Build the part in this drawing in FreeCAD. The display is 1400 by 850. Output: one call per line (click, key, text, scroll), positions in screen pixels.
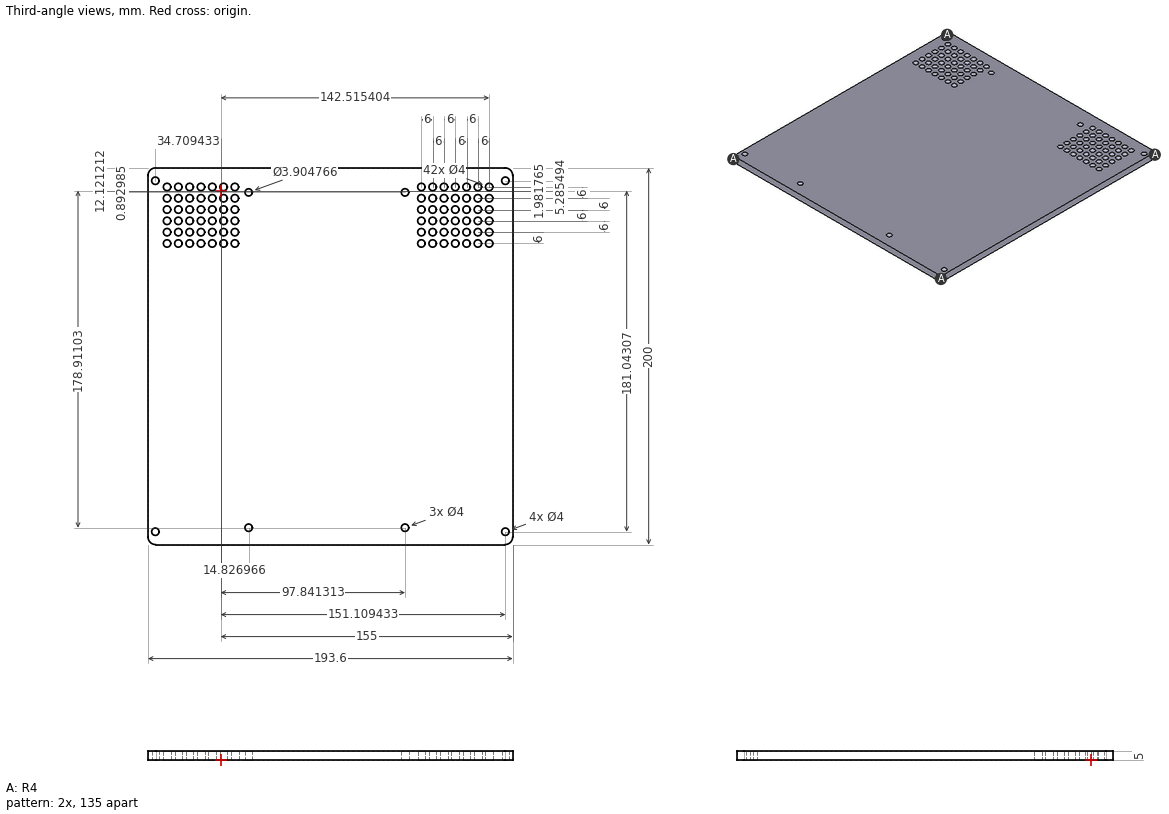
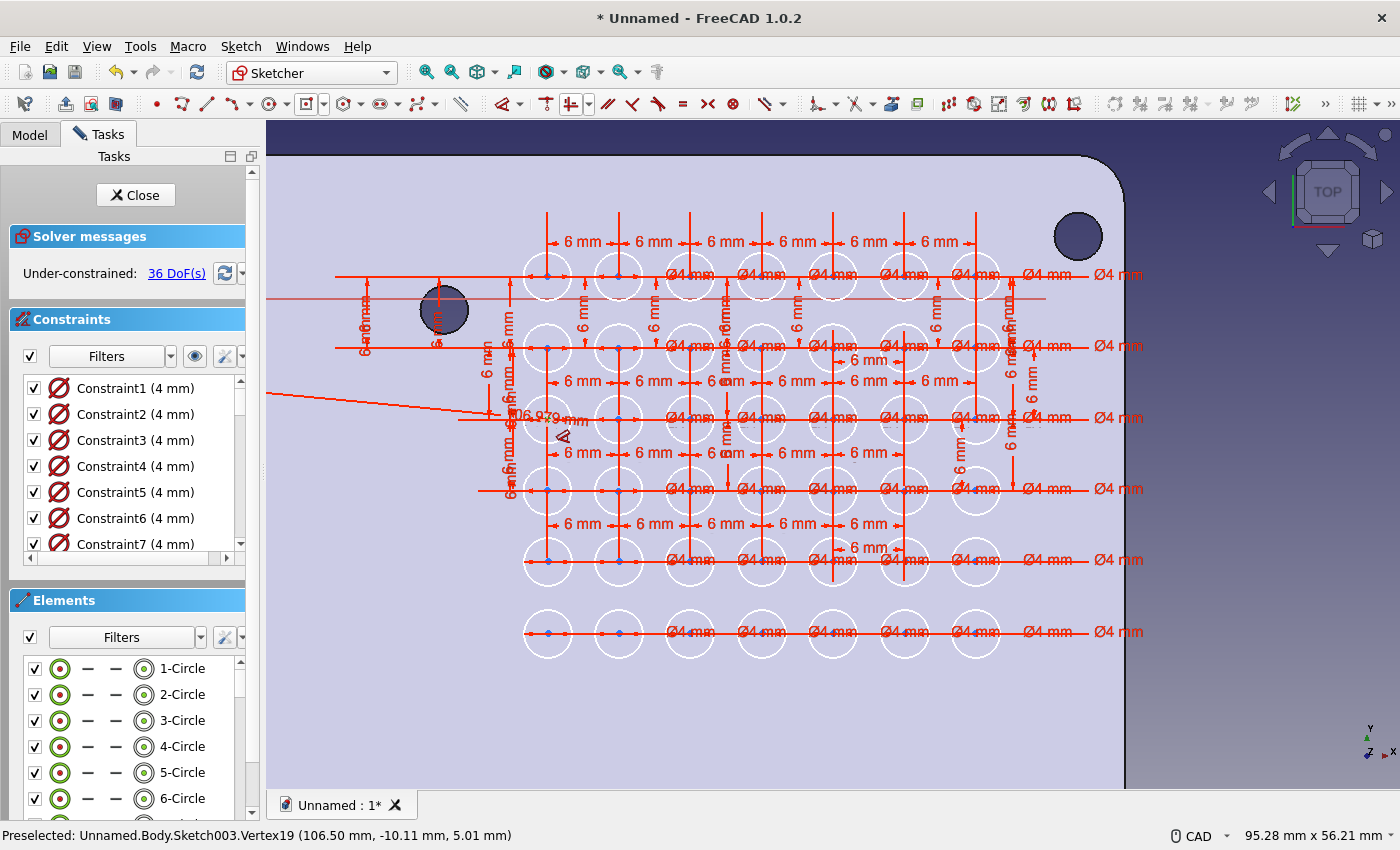
click(547, 491)
click(489, 430)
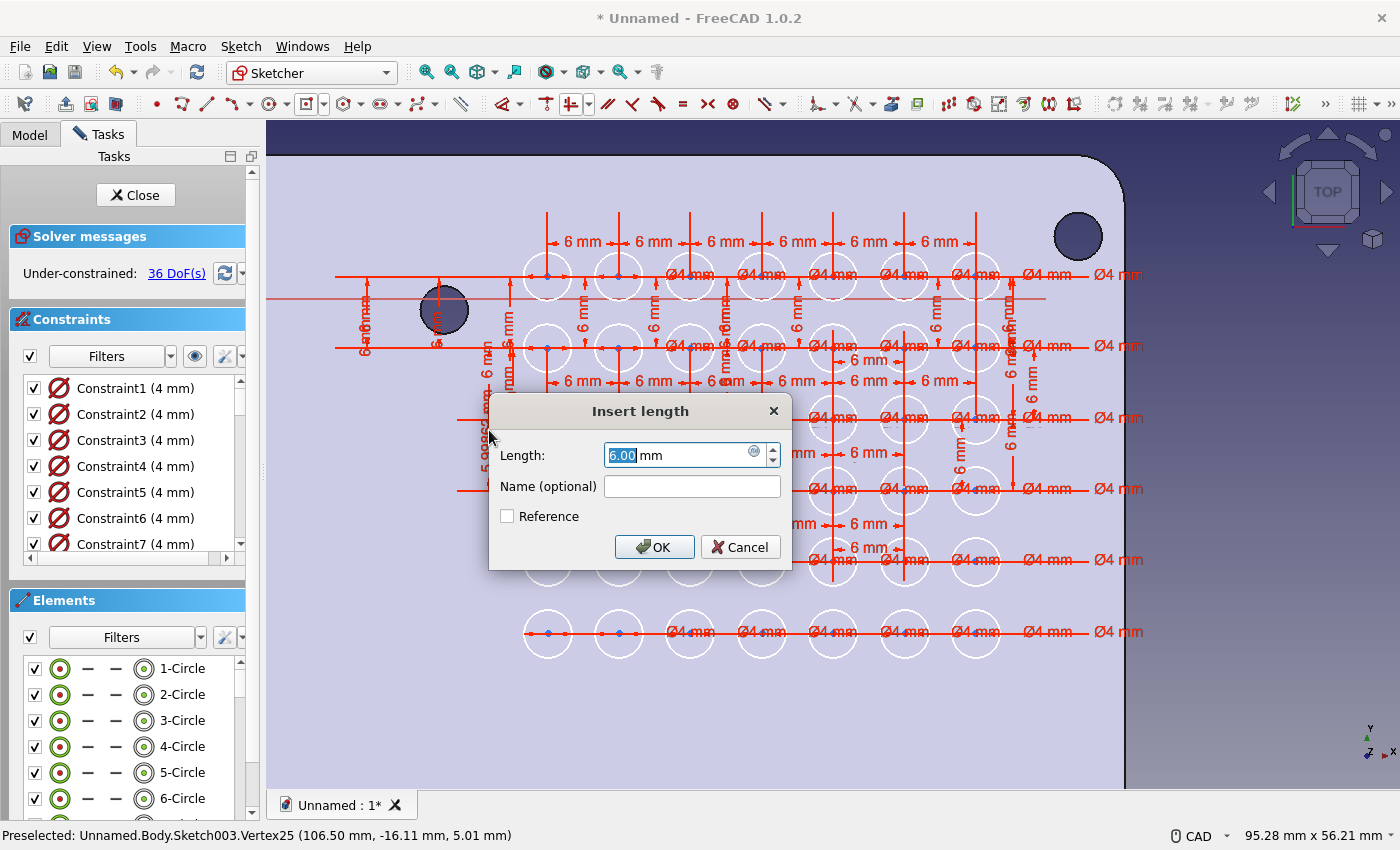
text(6)
key(Return)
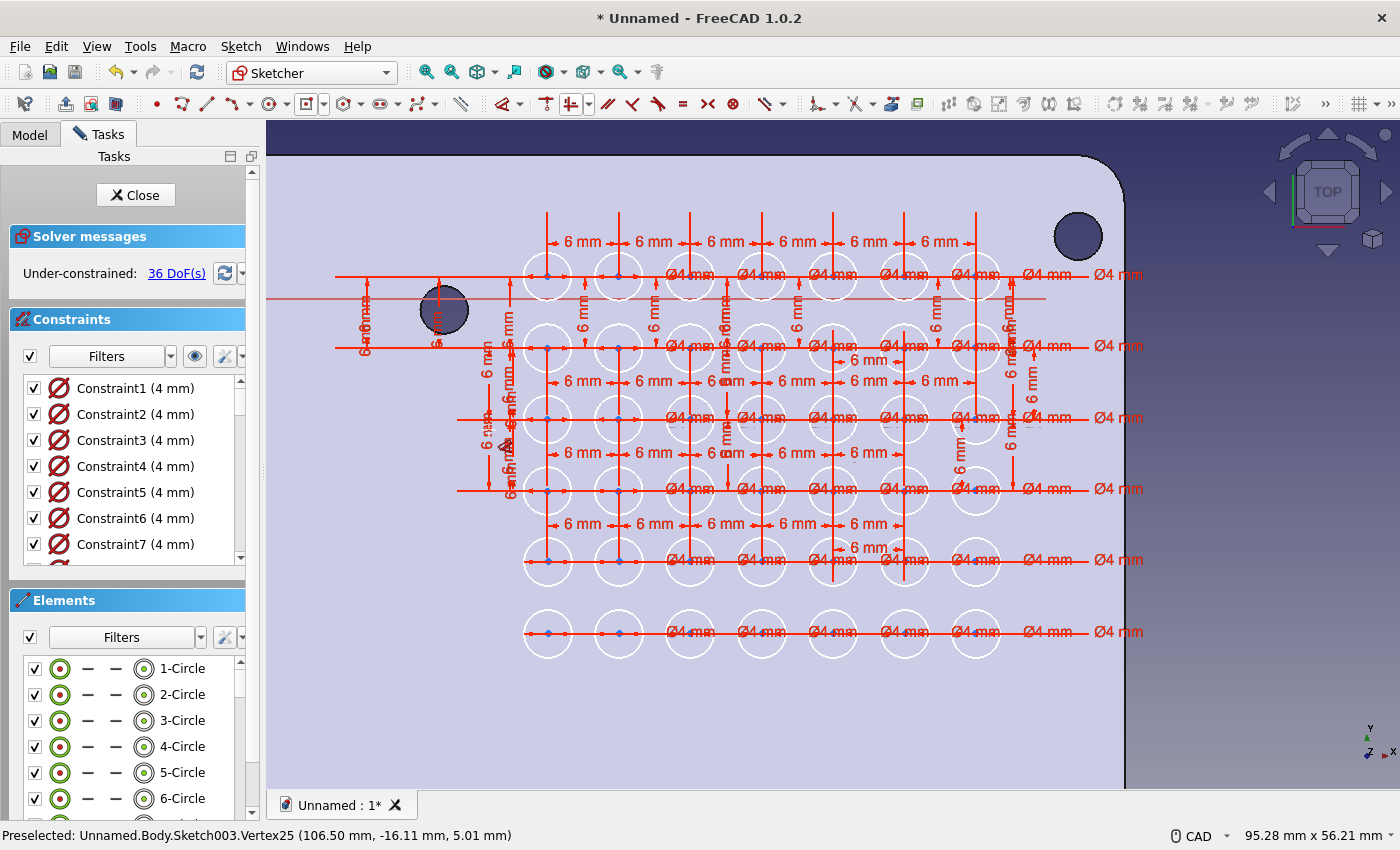
click(833, 491)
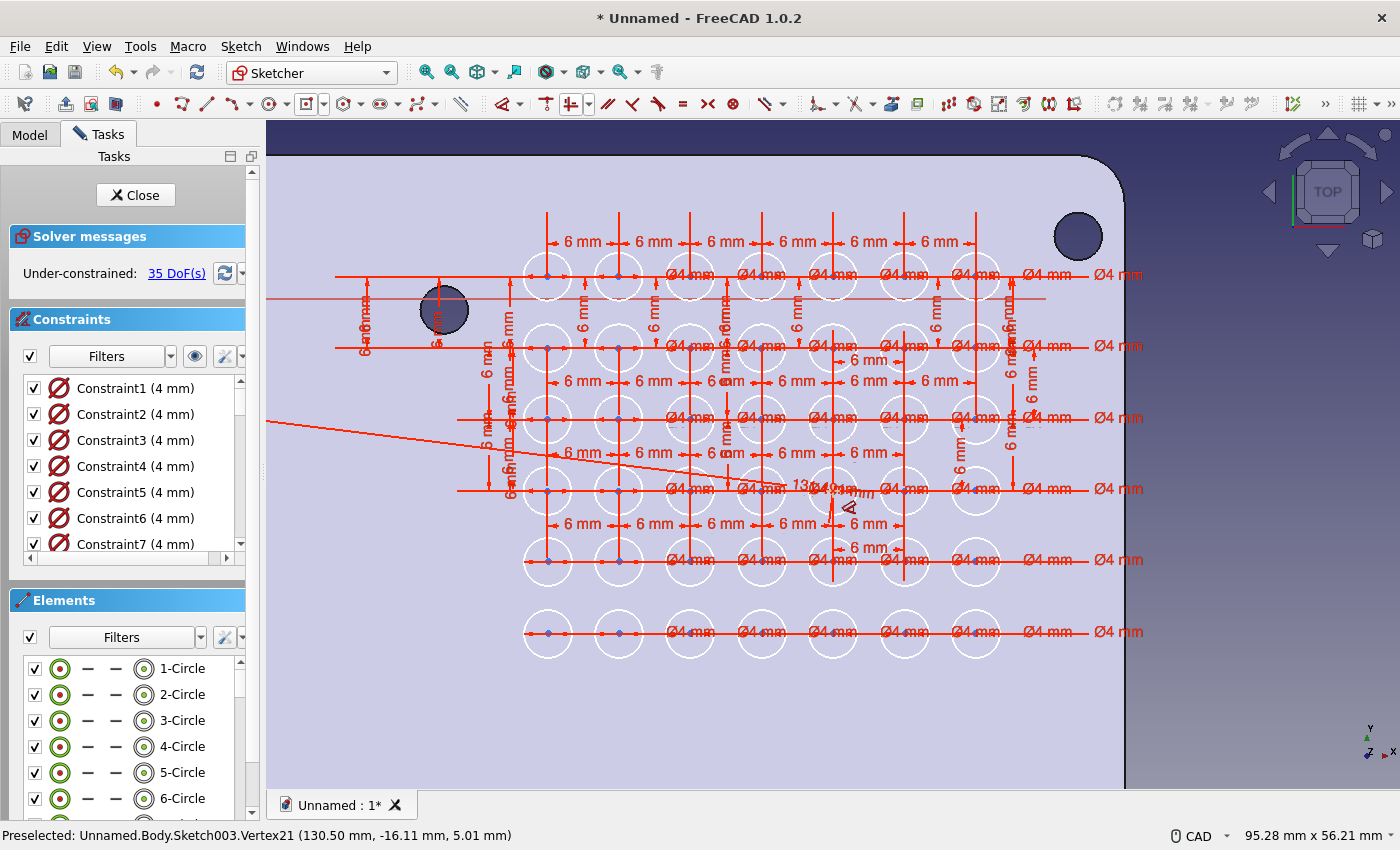
click(905, 562)
click(869, 596)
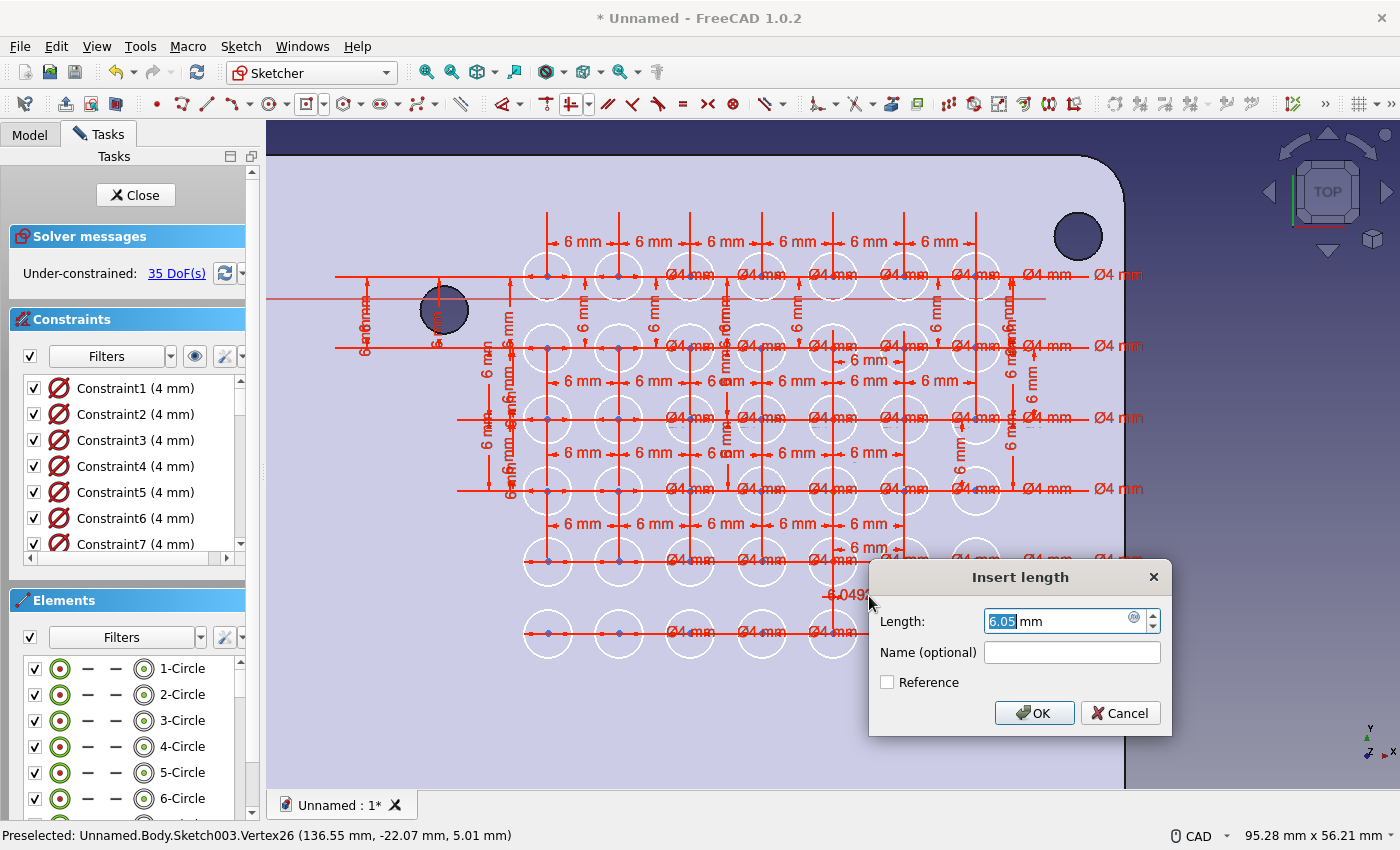
text(6)
key(Return)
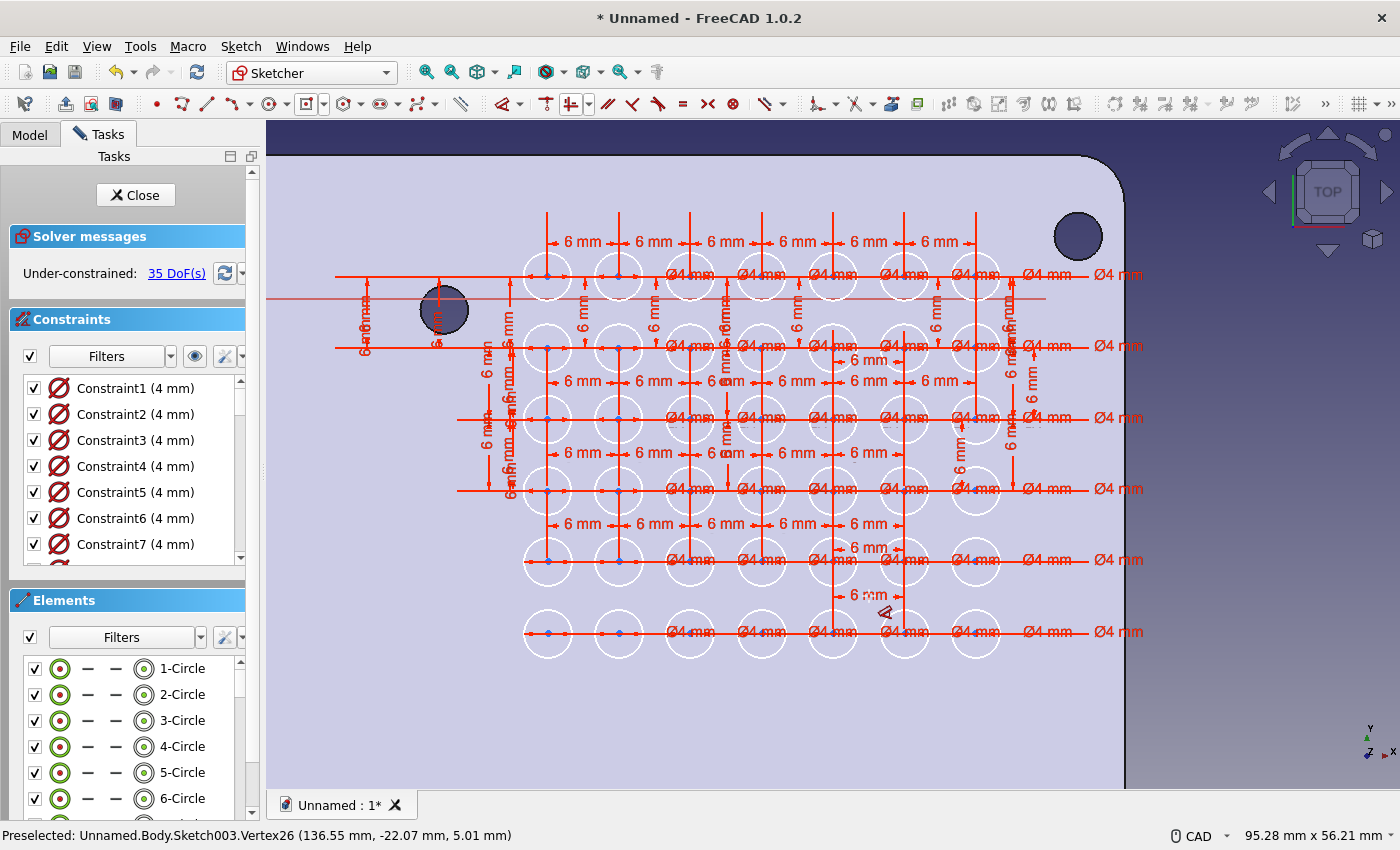
click(904, 491)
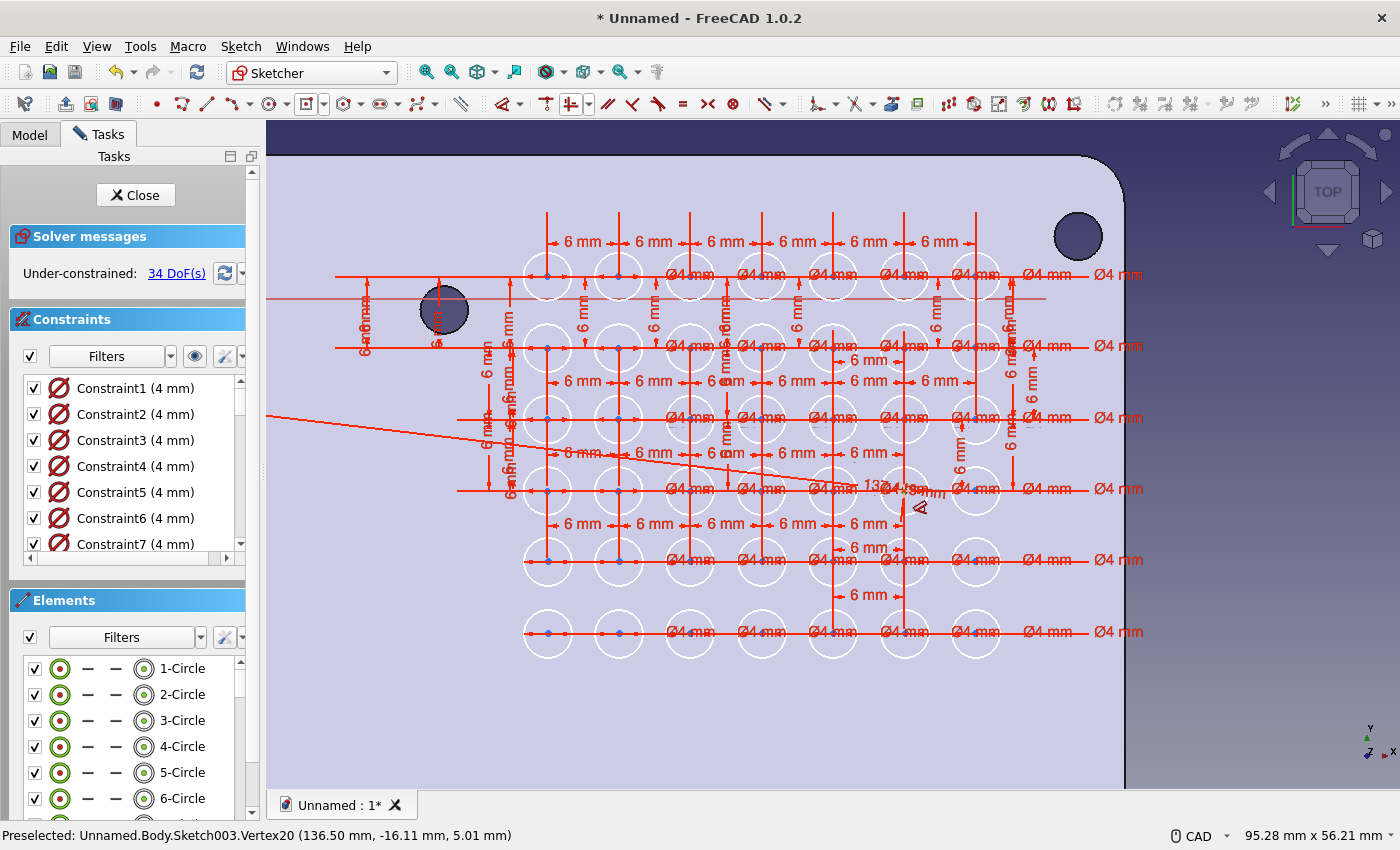
click(904, 562)
click(962, 527)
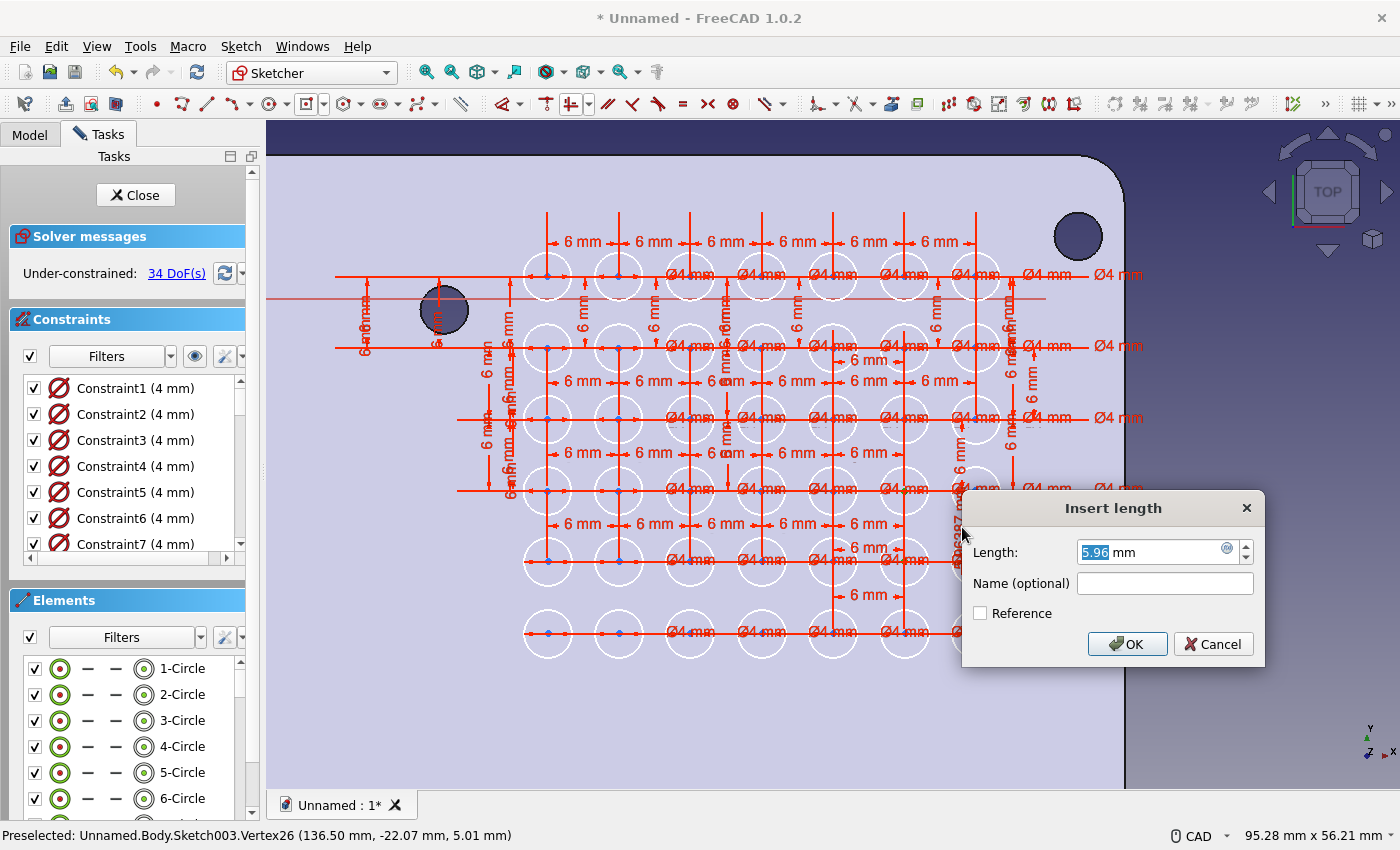
text(6)
key(Return)